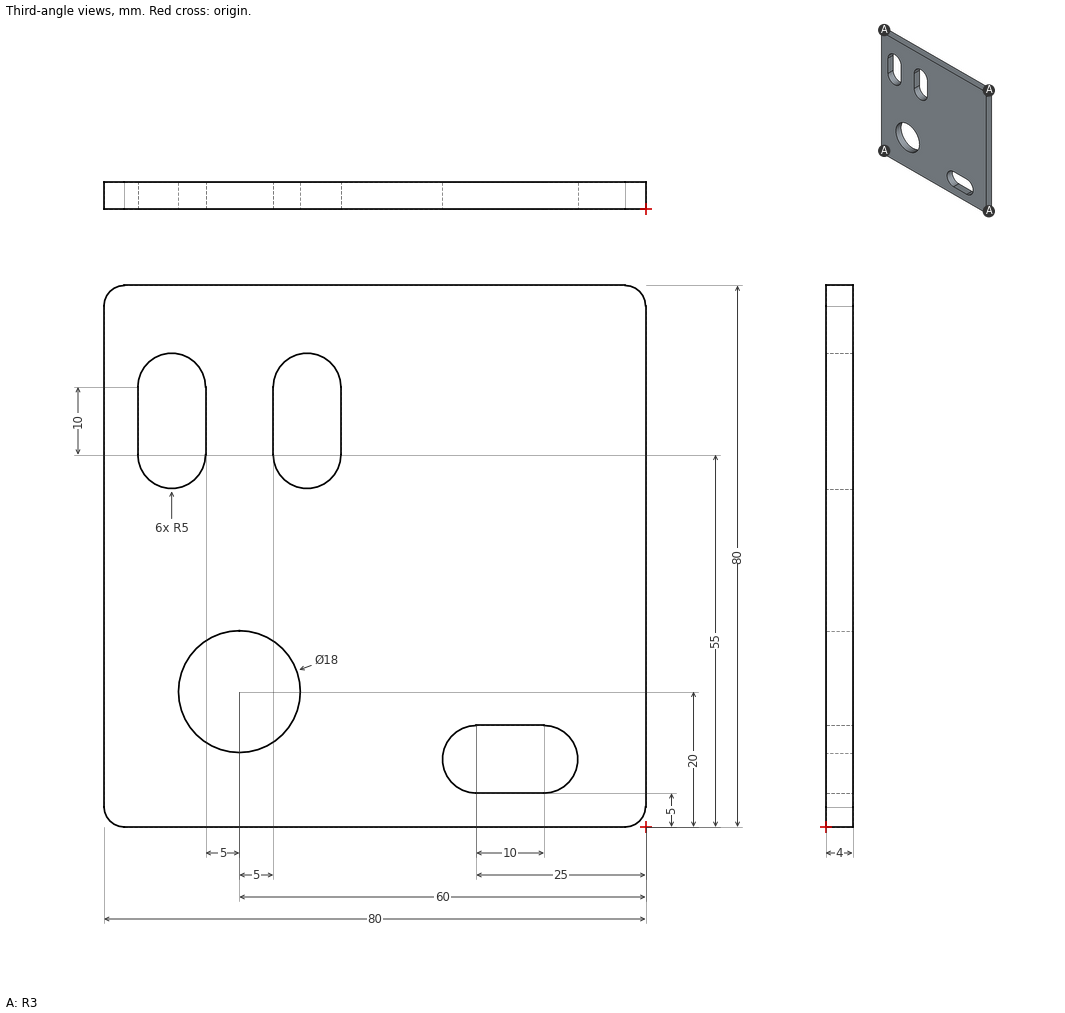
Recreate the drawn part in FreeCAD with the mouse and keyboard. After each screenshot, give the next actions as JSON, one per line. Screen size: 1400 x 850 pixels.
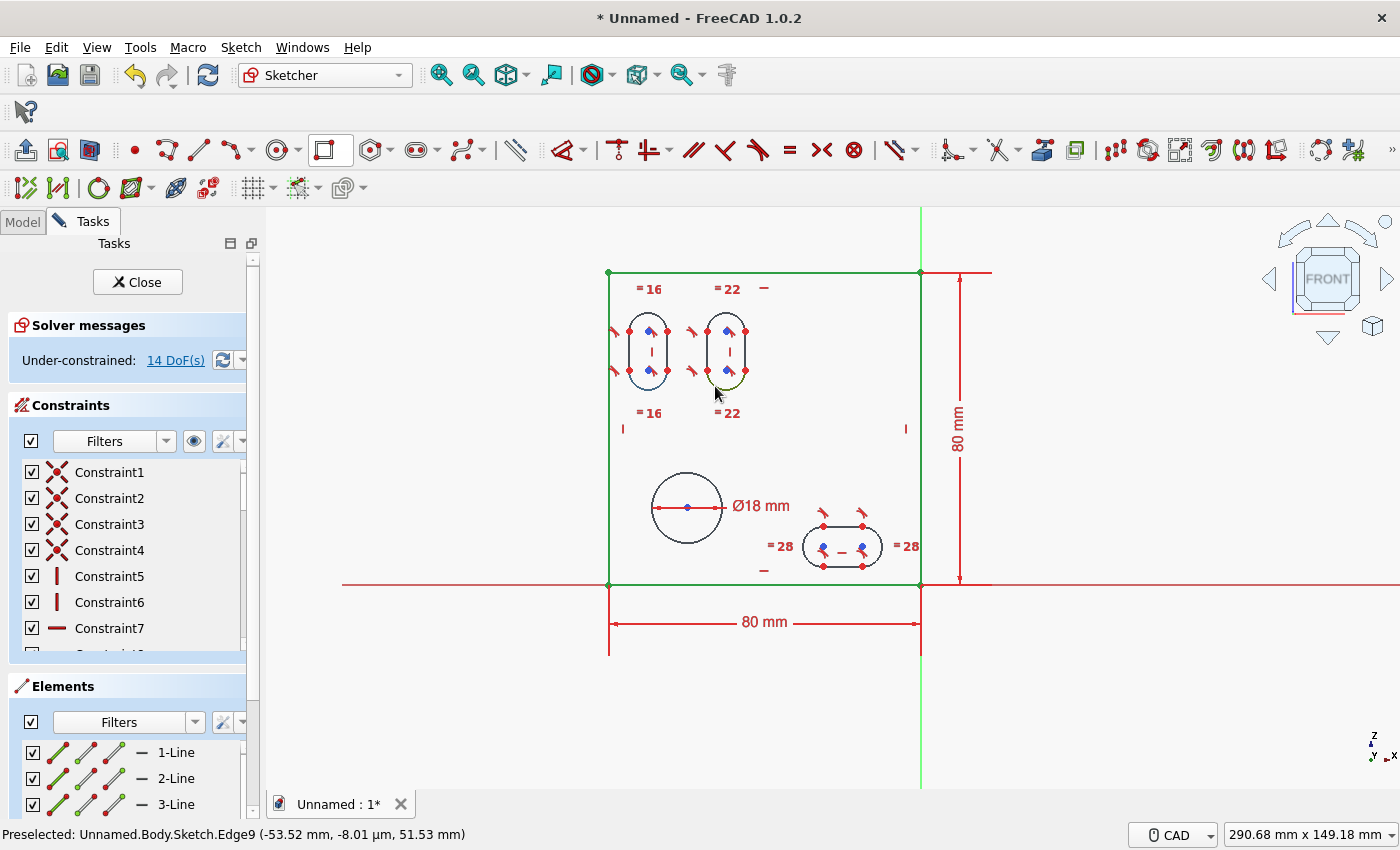
{"action": "left_click", "coordinate": [807, 535]}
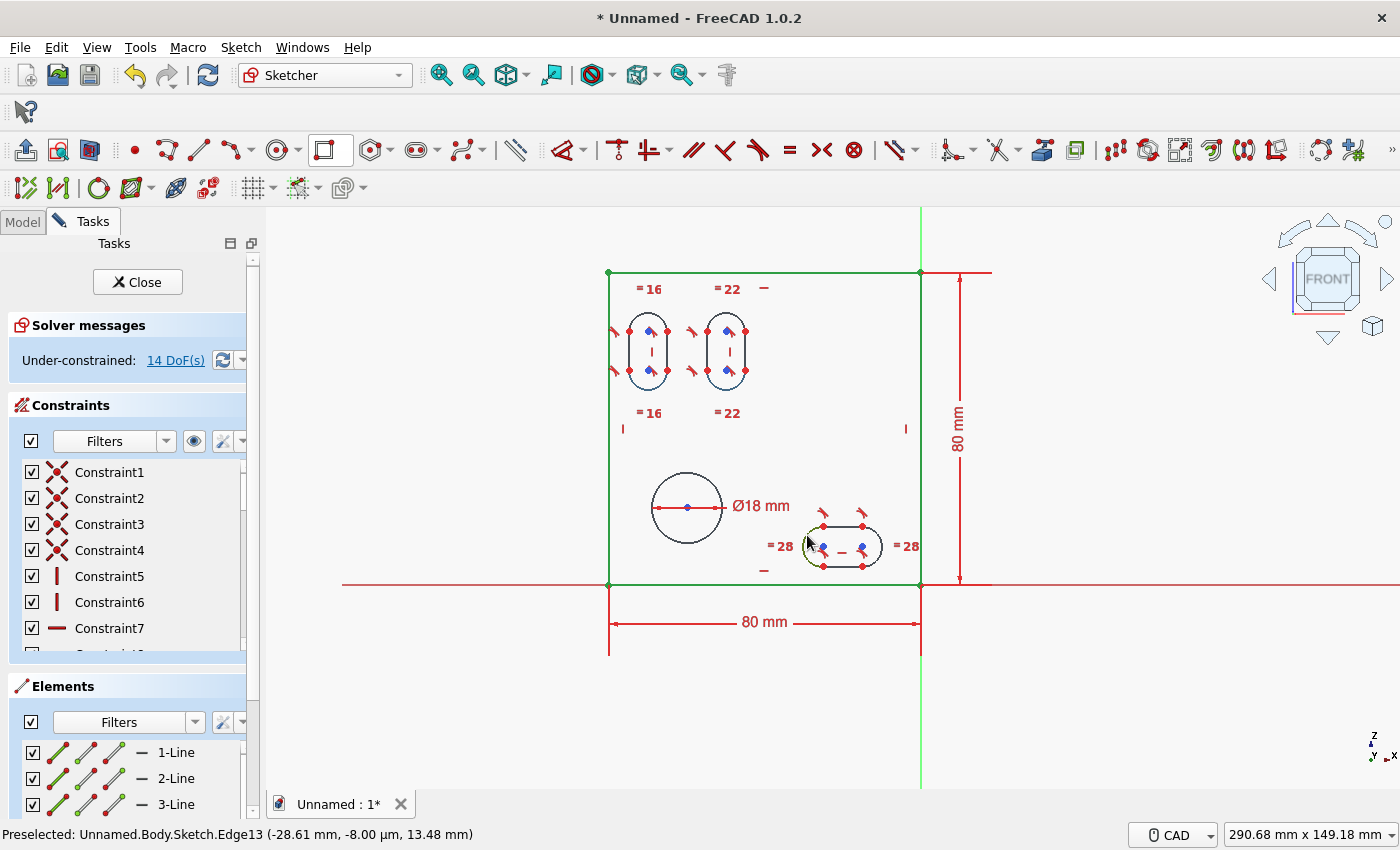
{"action": "left_click", "coordinate": [790, 150]}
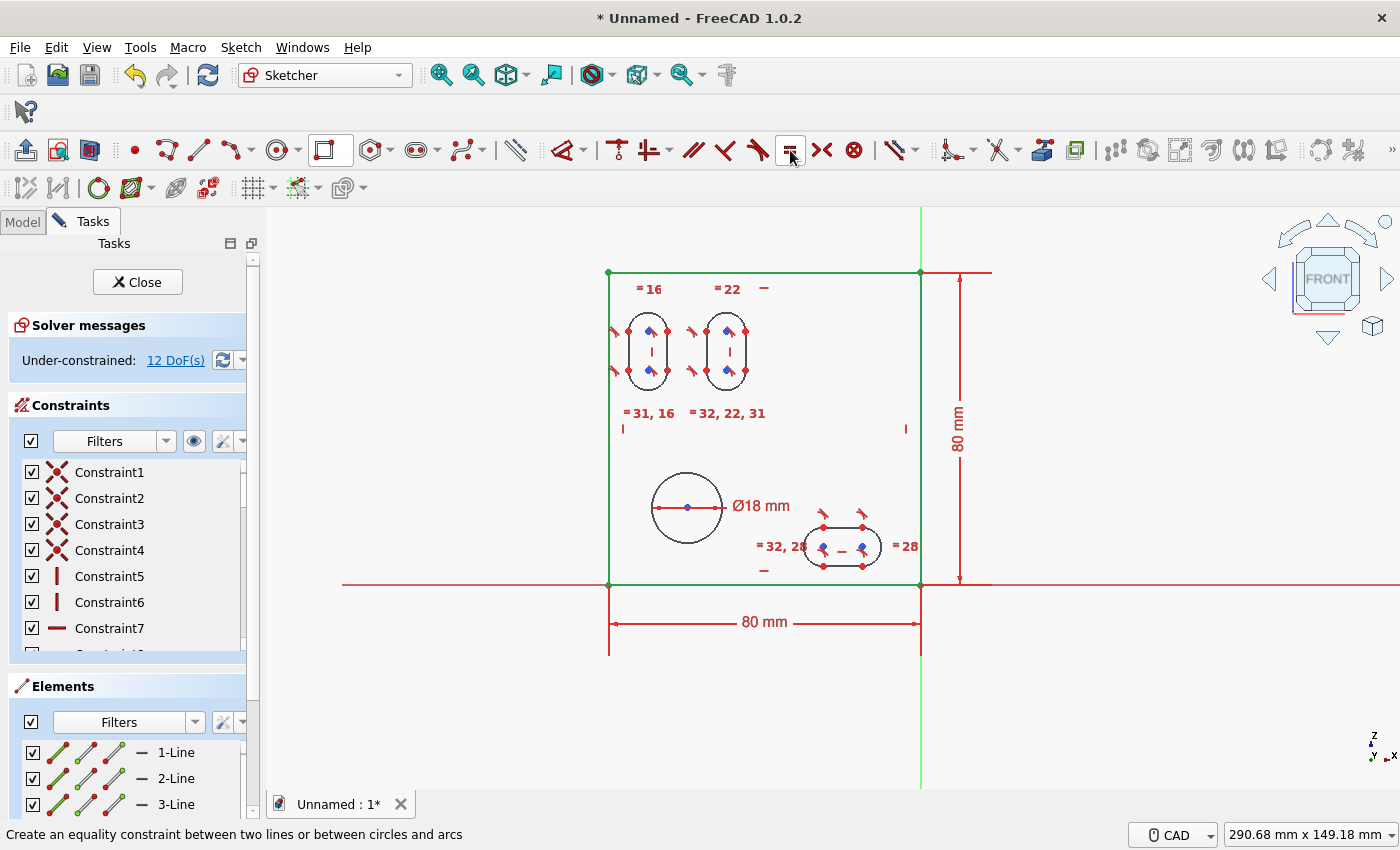
{"action": "left_click", "coordinate": [562, 150]}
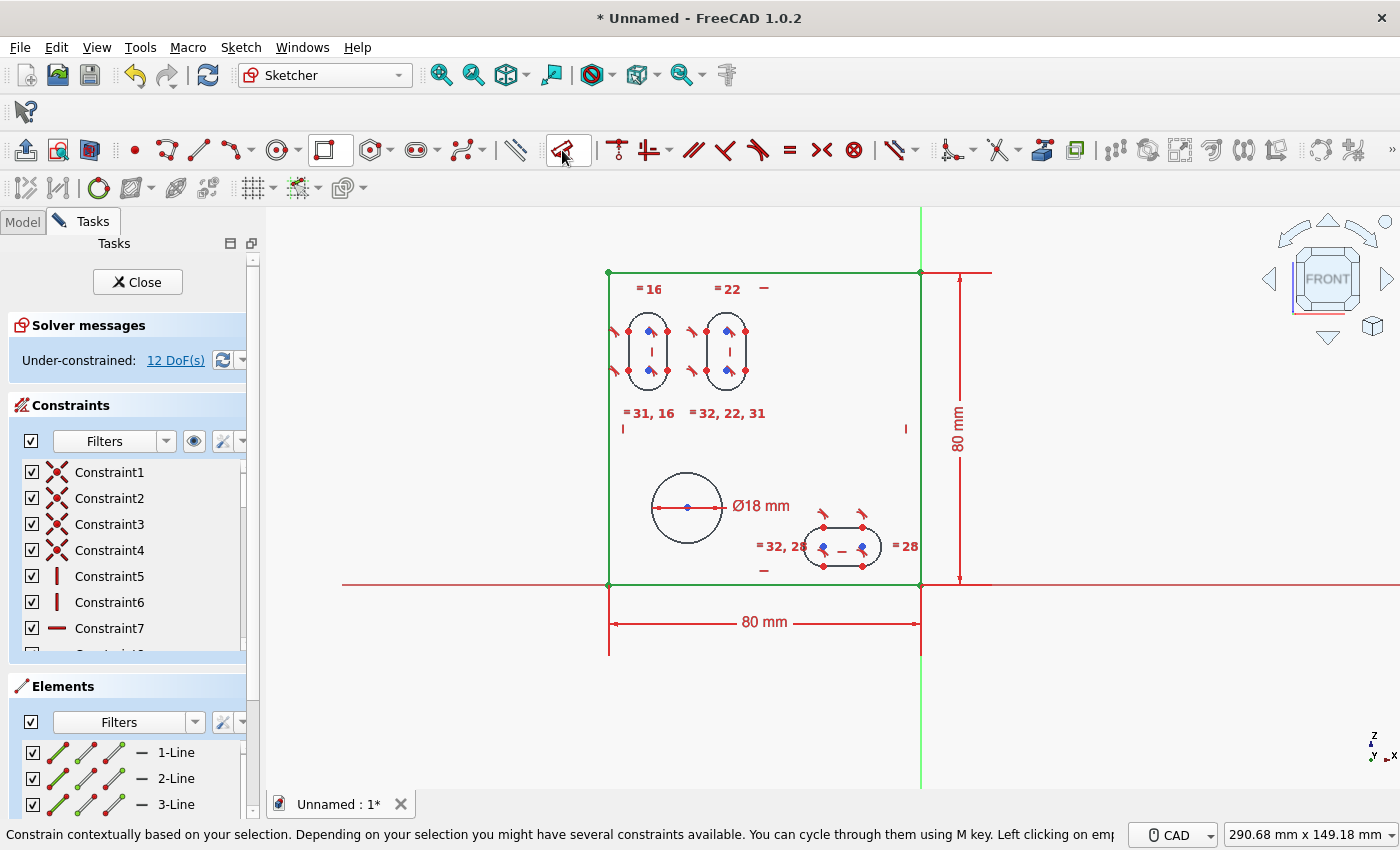
{"action": "scroll", "coordinate": [637, 387], "scroll_direction": "up", "scroll_amount": 4}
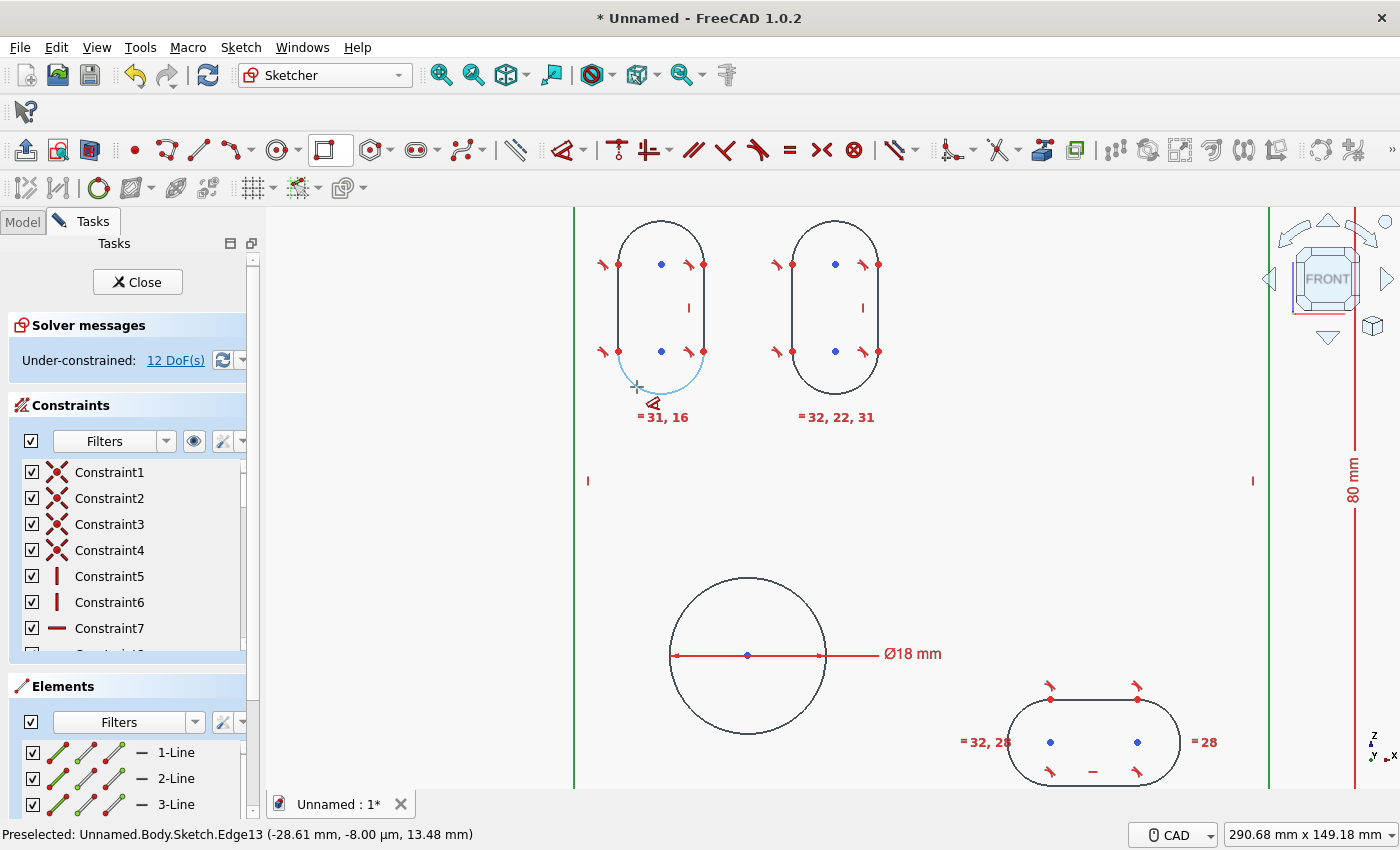
{"action": "left_click", "coordinate": [636, 386]}
{"action": "left_click", "coordinate": [617, 412]}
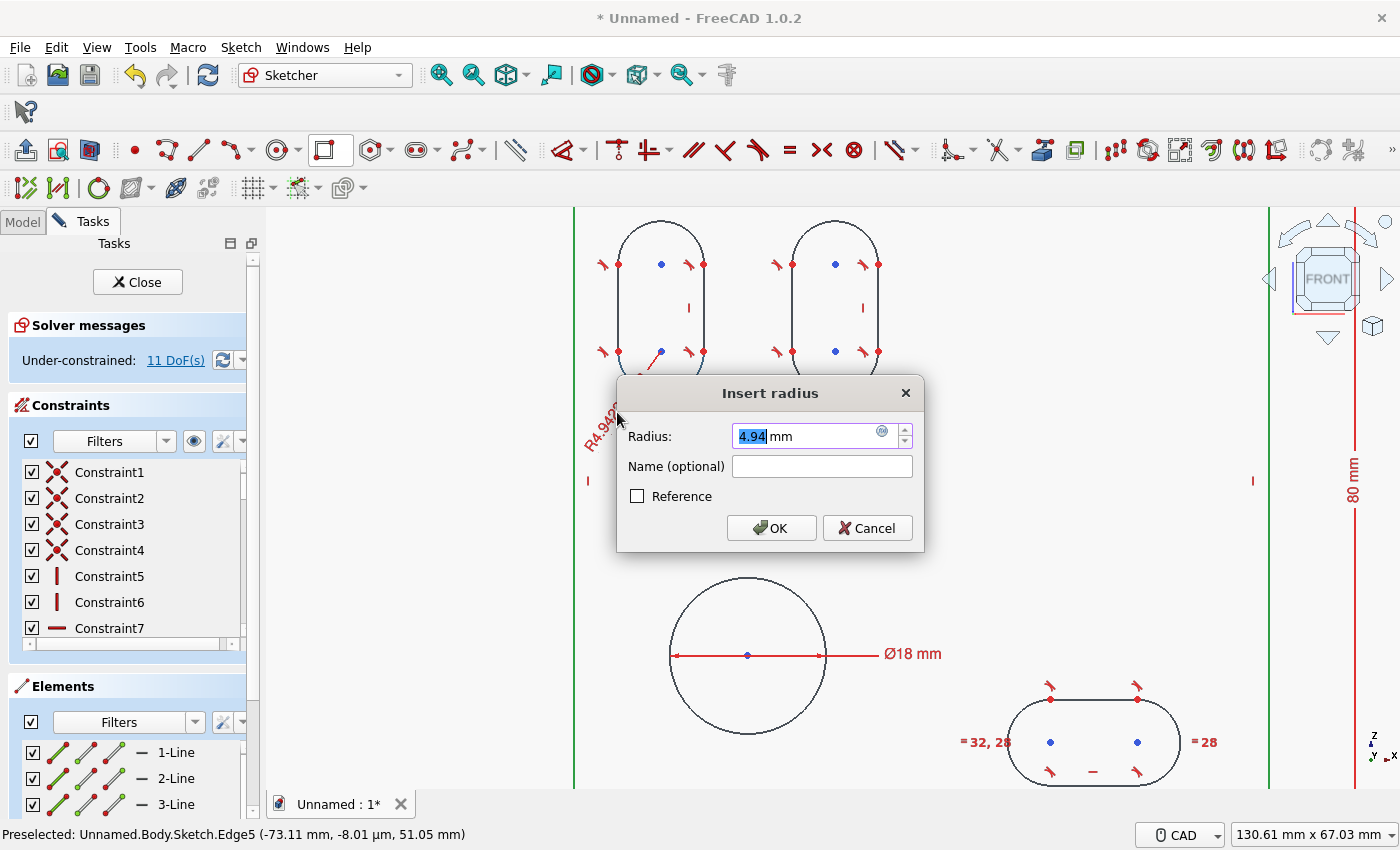
{"action": "type", "text": "5"}
{"action": "key", "text": "Return"}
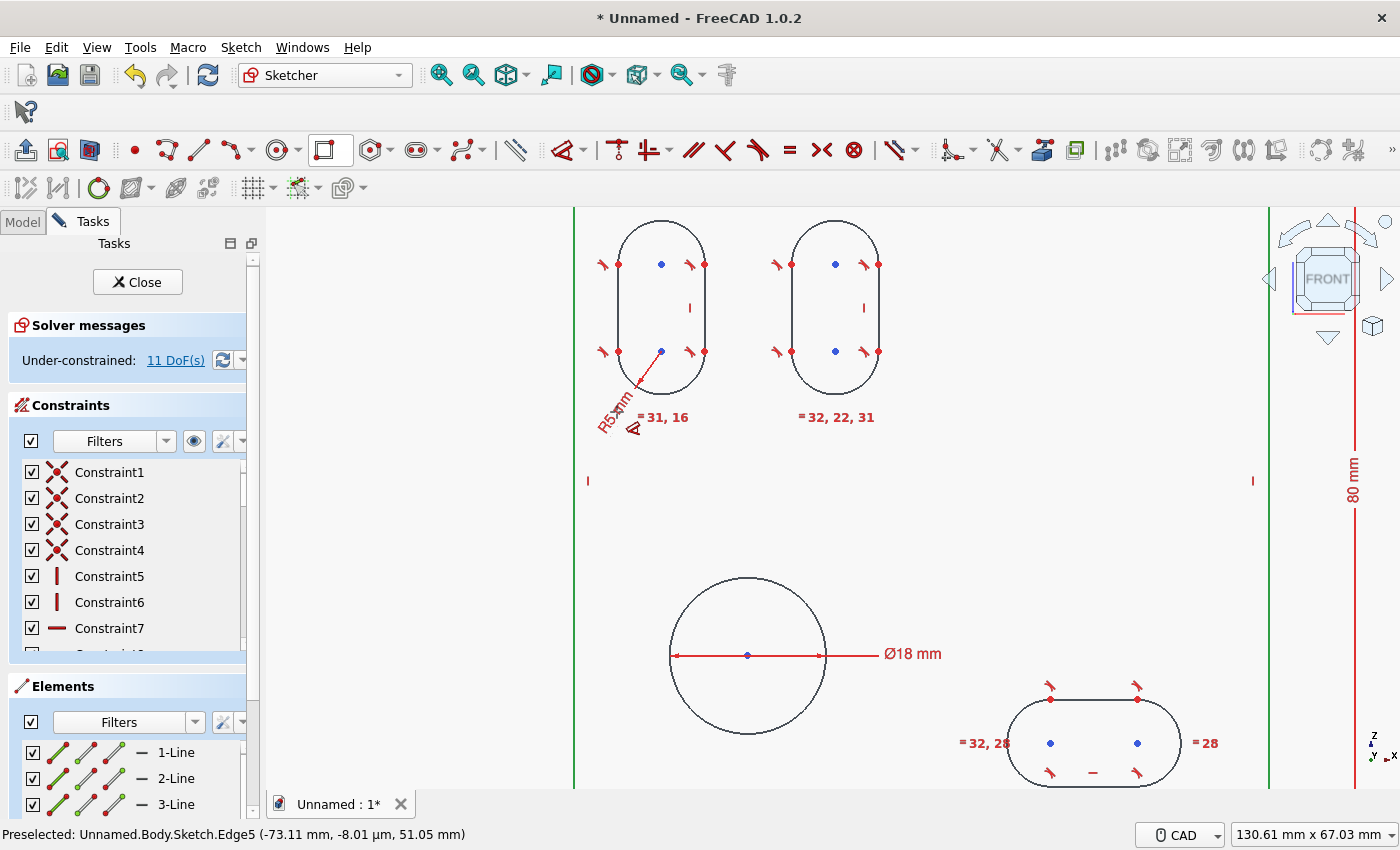
{"action": "left_click", "coordinate": [618, 325]}
{"action": "left_click", "coordinate": [652, 308]}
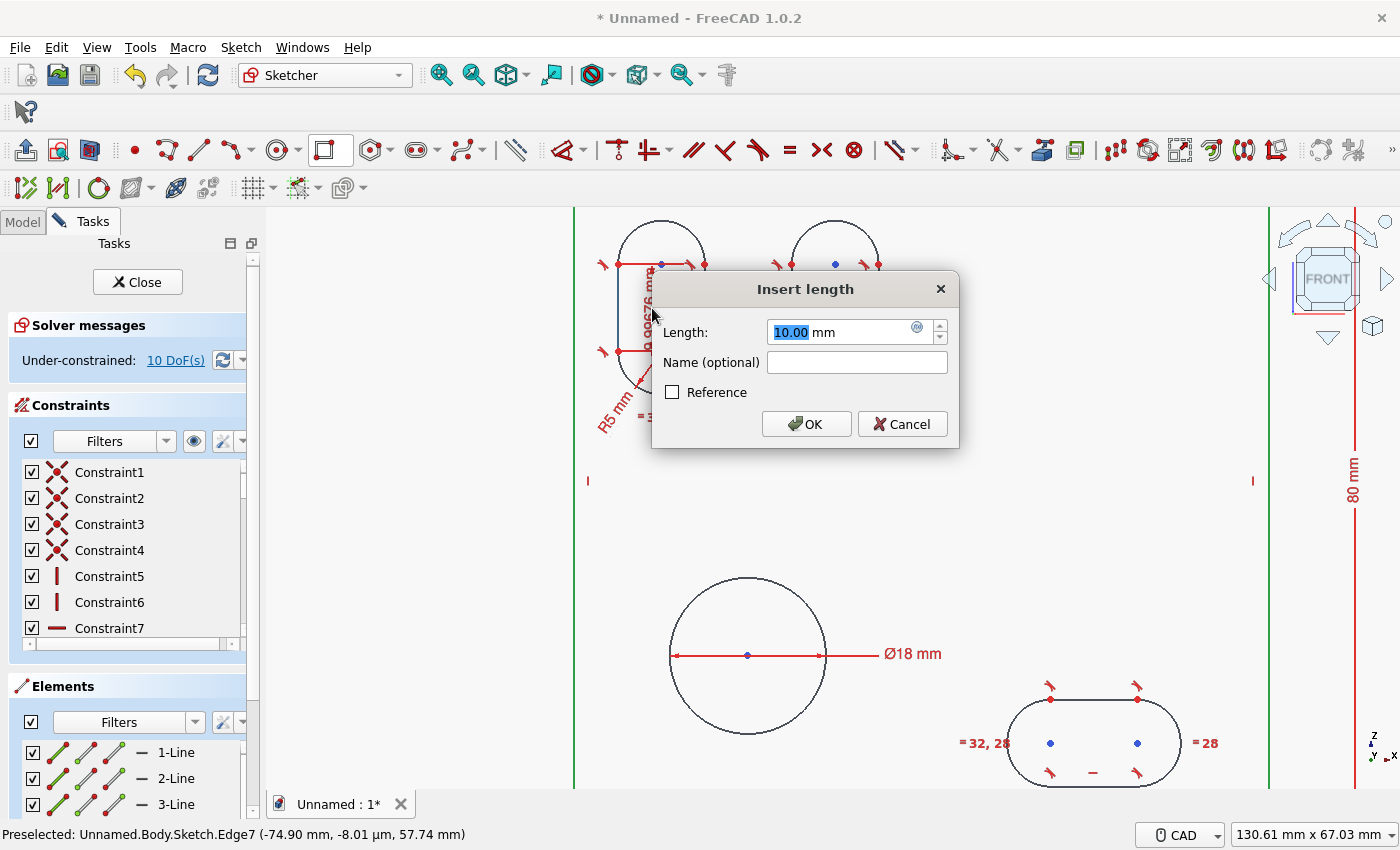
{"action": "type", "text": "10"}
{"action": "key", "text": "Return"}